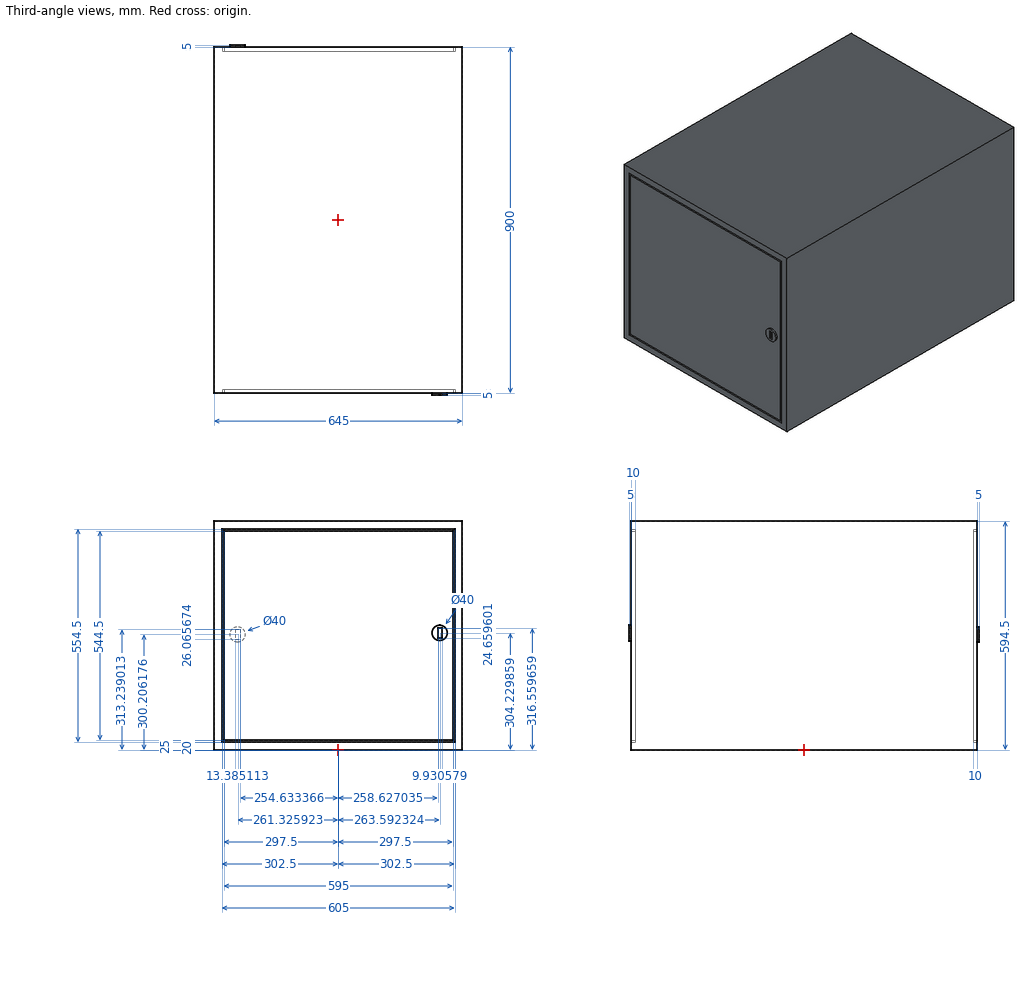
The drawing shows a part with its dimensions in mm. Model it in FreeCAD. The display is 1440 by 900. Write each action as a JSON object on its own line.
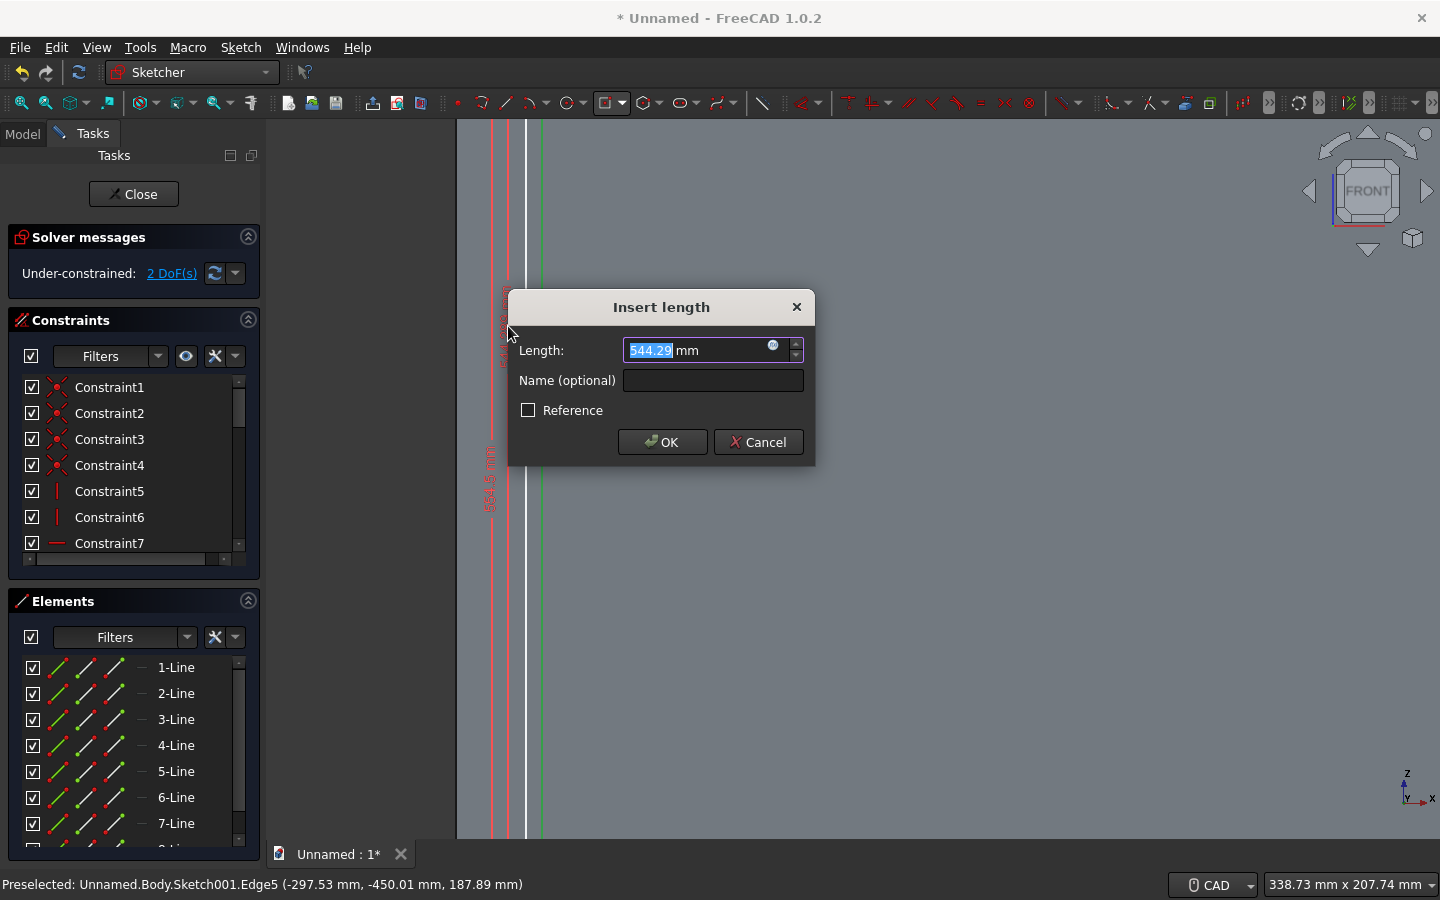
{"action": "type", "text": "544.5"}
{"action": "key", "text": "Return"}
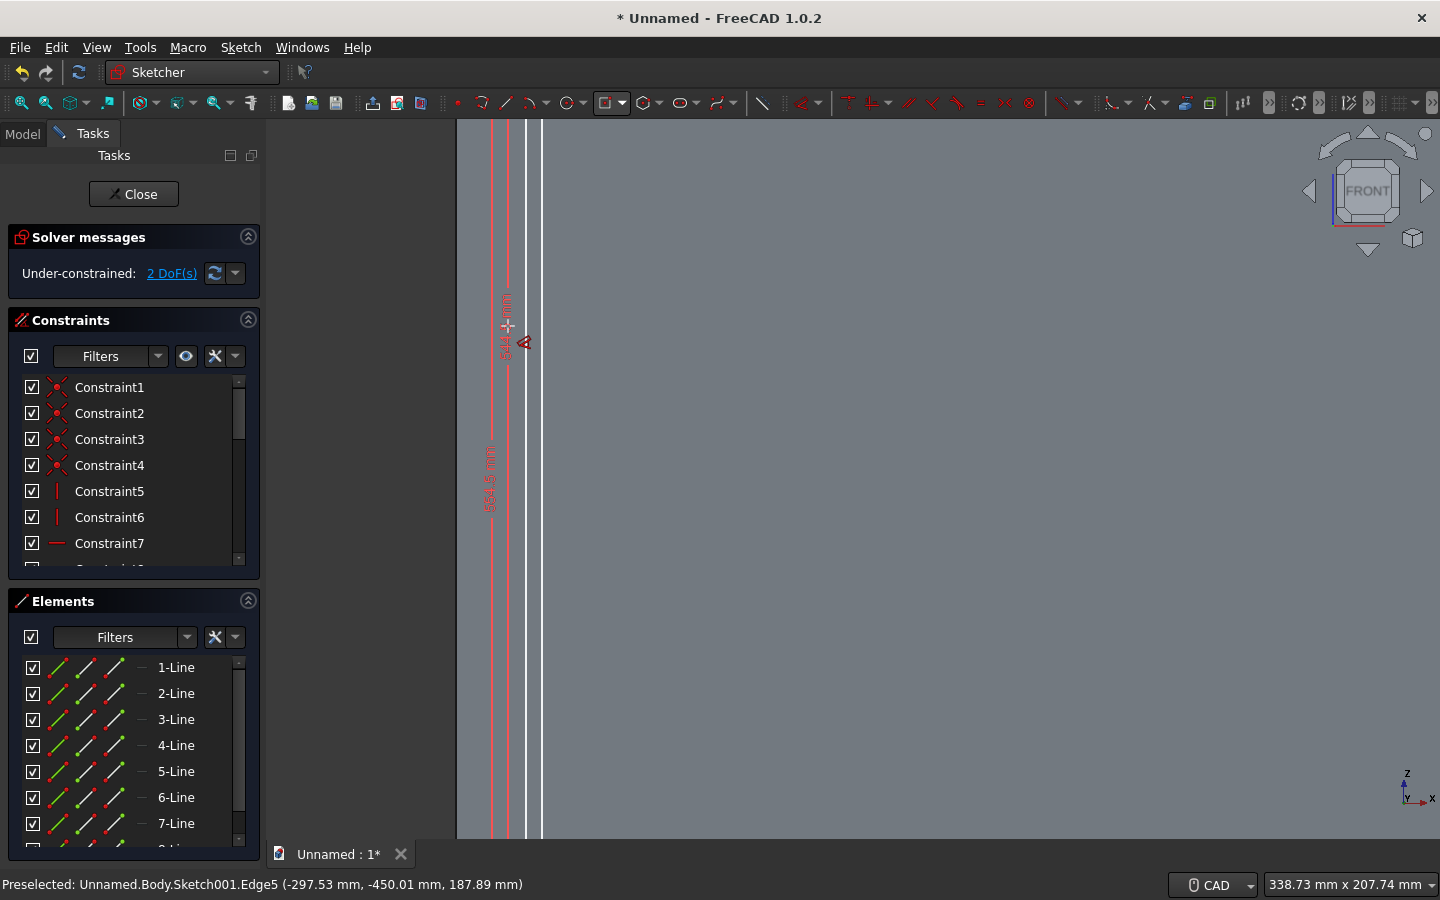
{"action": "scroll", "coordinate": [526, 646], "scroll_direction": "down", "scroll_amount": 7}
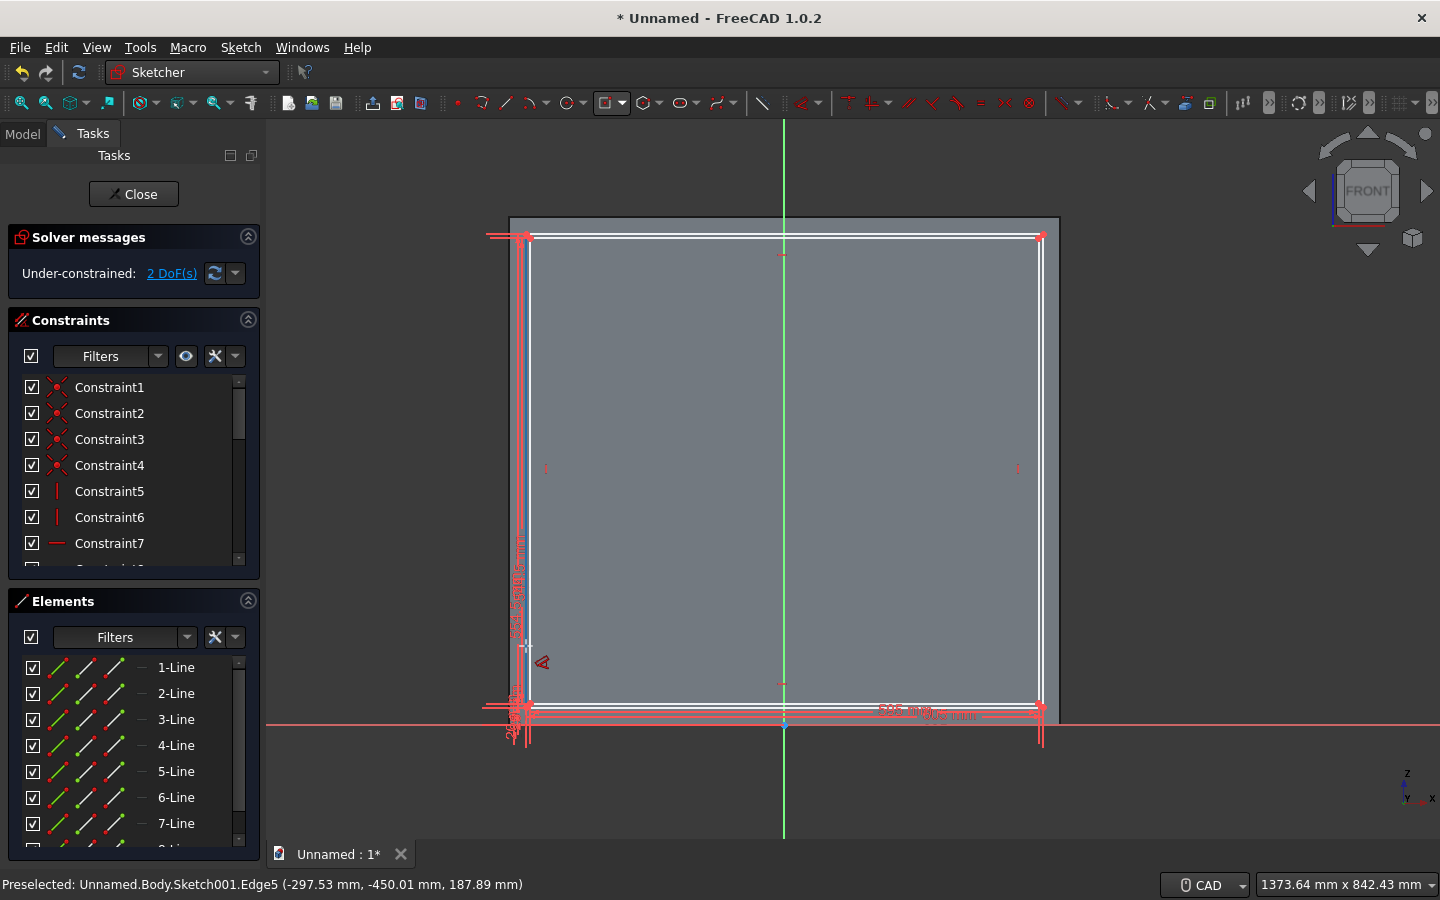
{"action": "scroll", "coordinate": [526, 234], "scroll_direction": "up", "scroll_amount": 4}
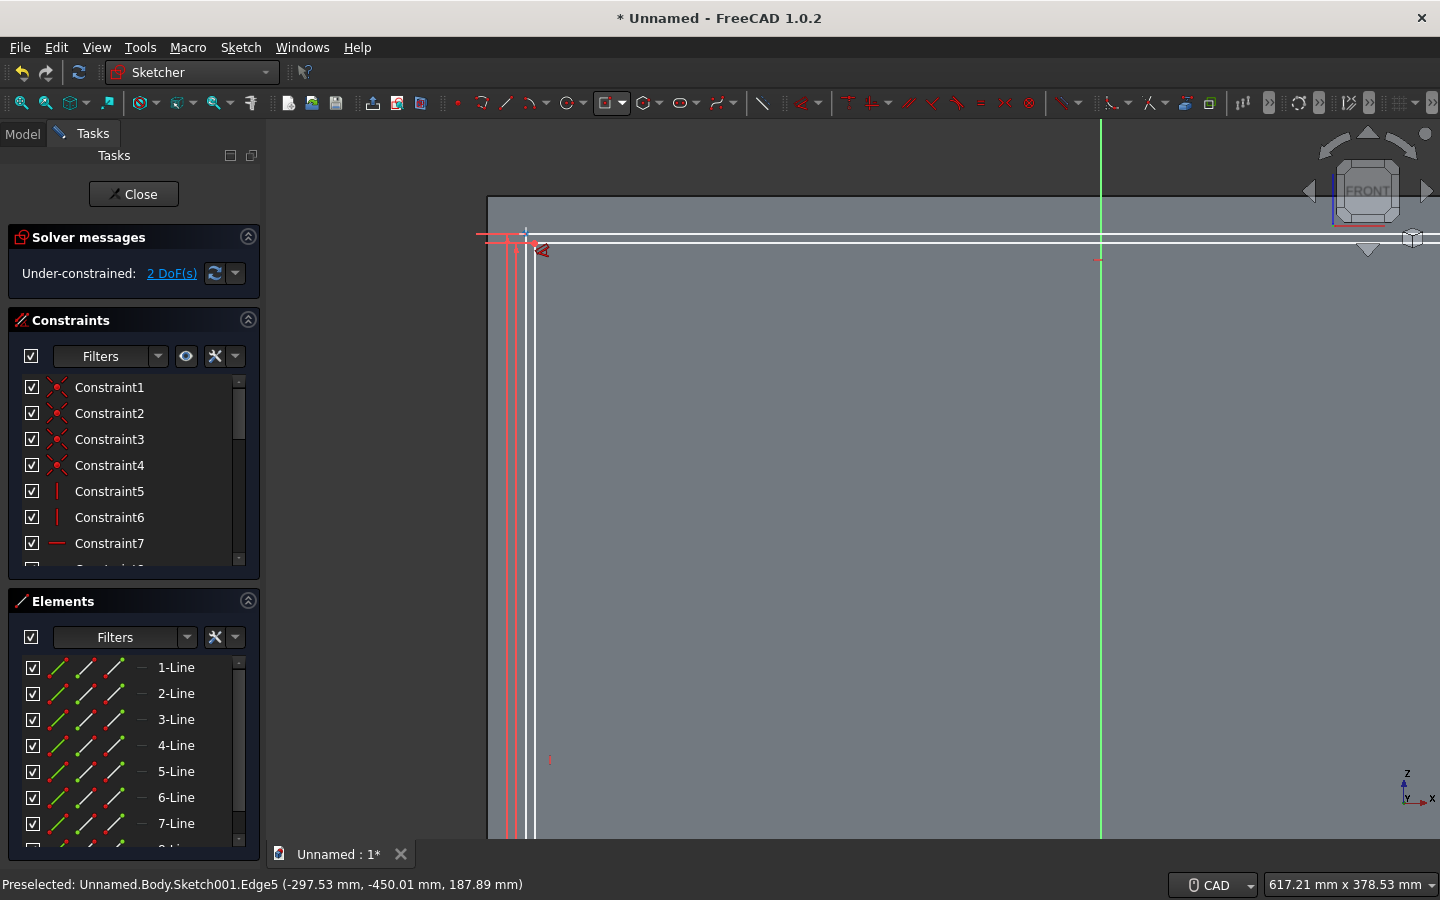
{"action": "left_click", "coordinate": [526, 234]}
{"action": "left_click", "coordinate": [813, 200]}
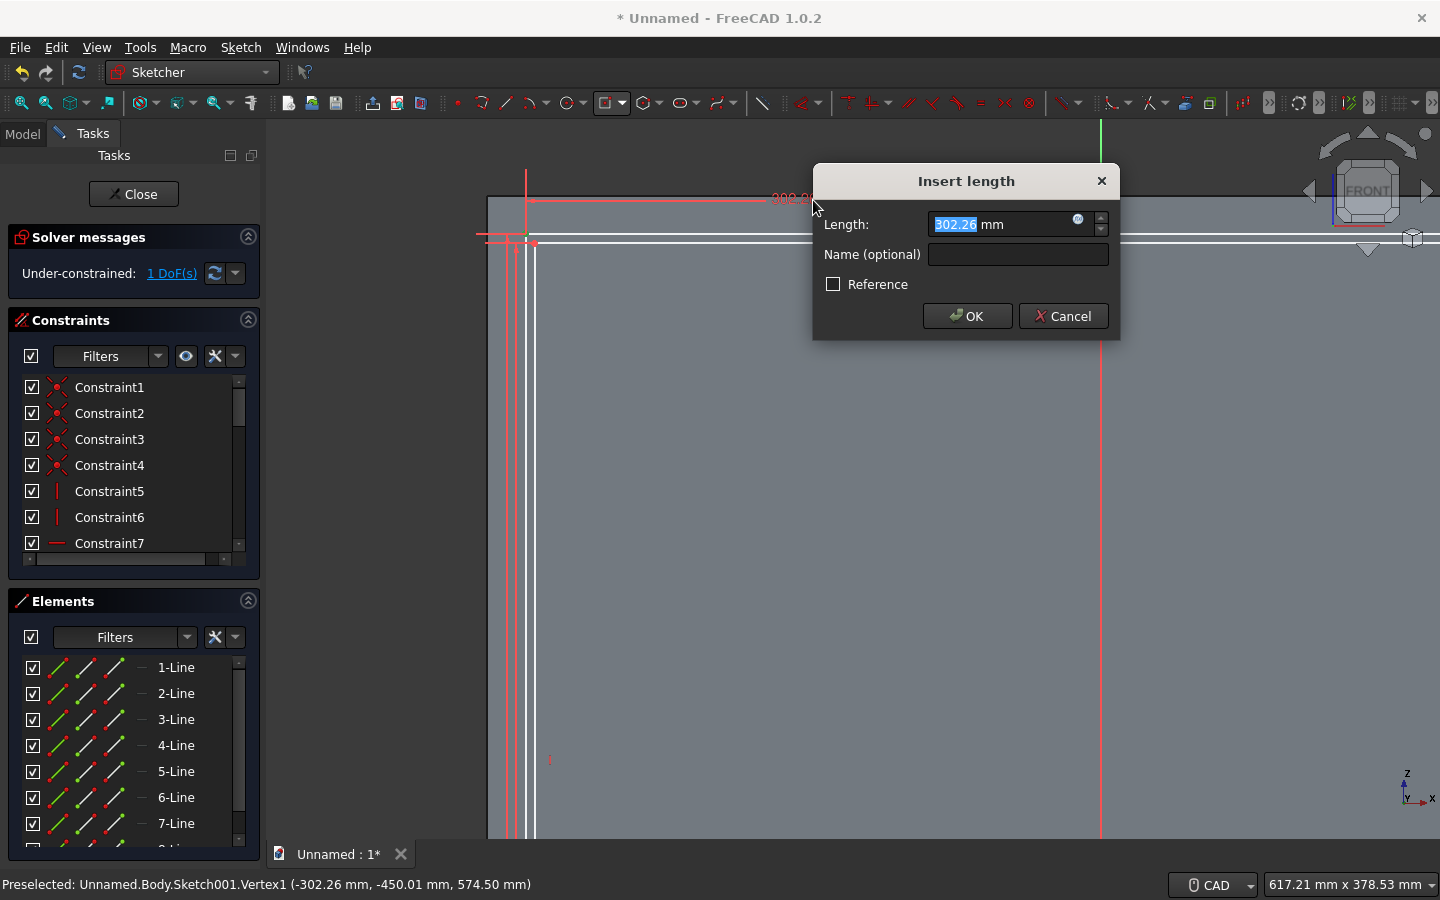
{"action": "type", "text": "302.5"}
{"action": "key", "text": "Return"}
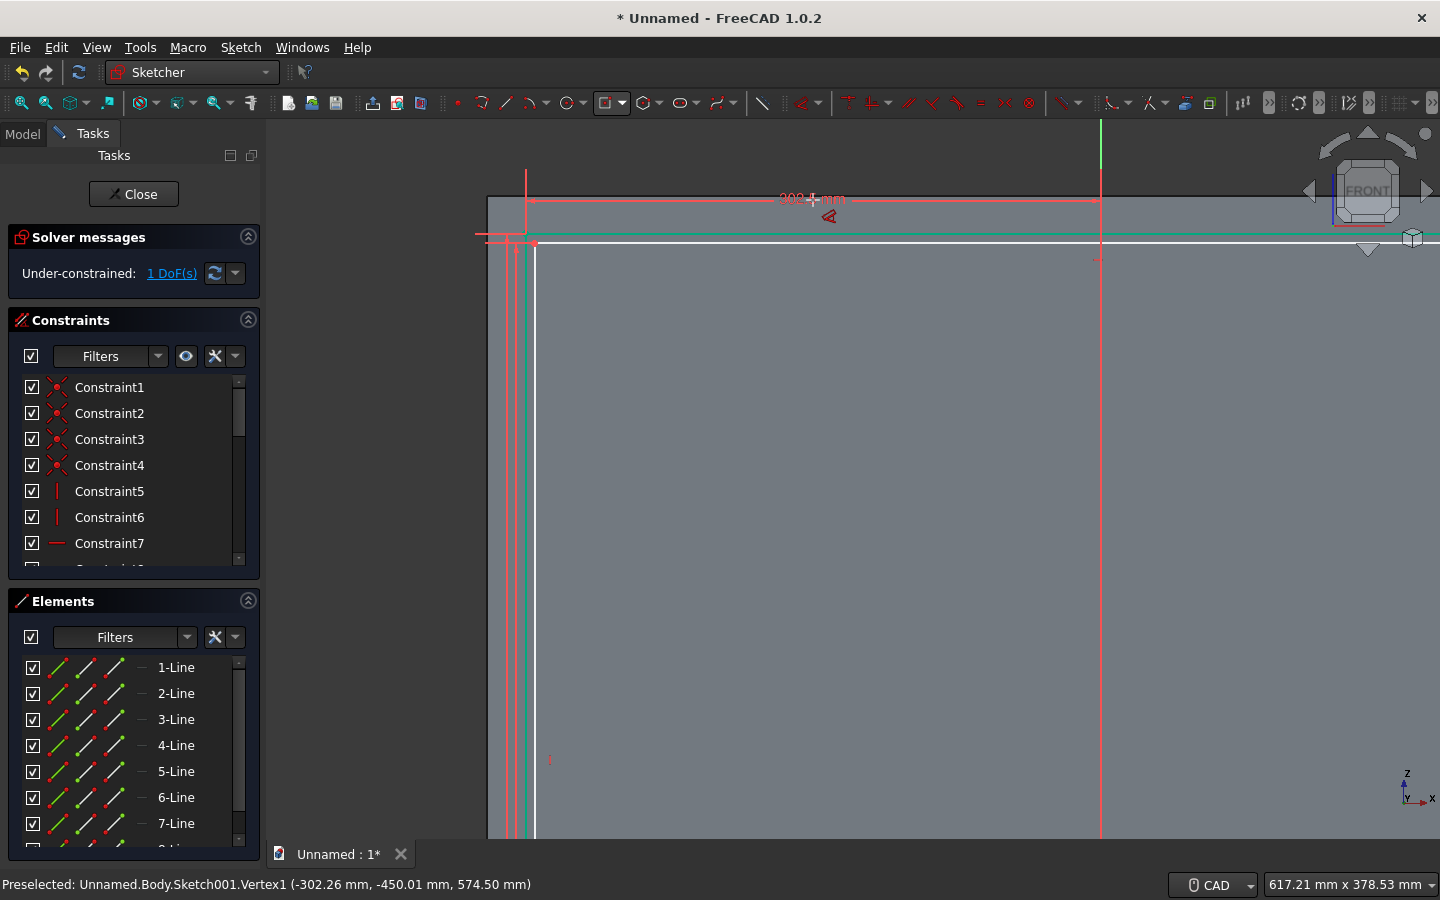
{"action": "left_click", "coordinate": [535, 243]}
{"action": "left_click", "coordinate": [688, 209]}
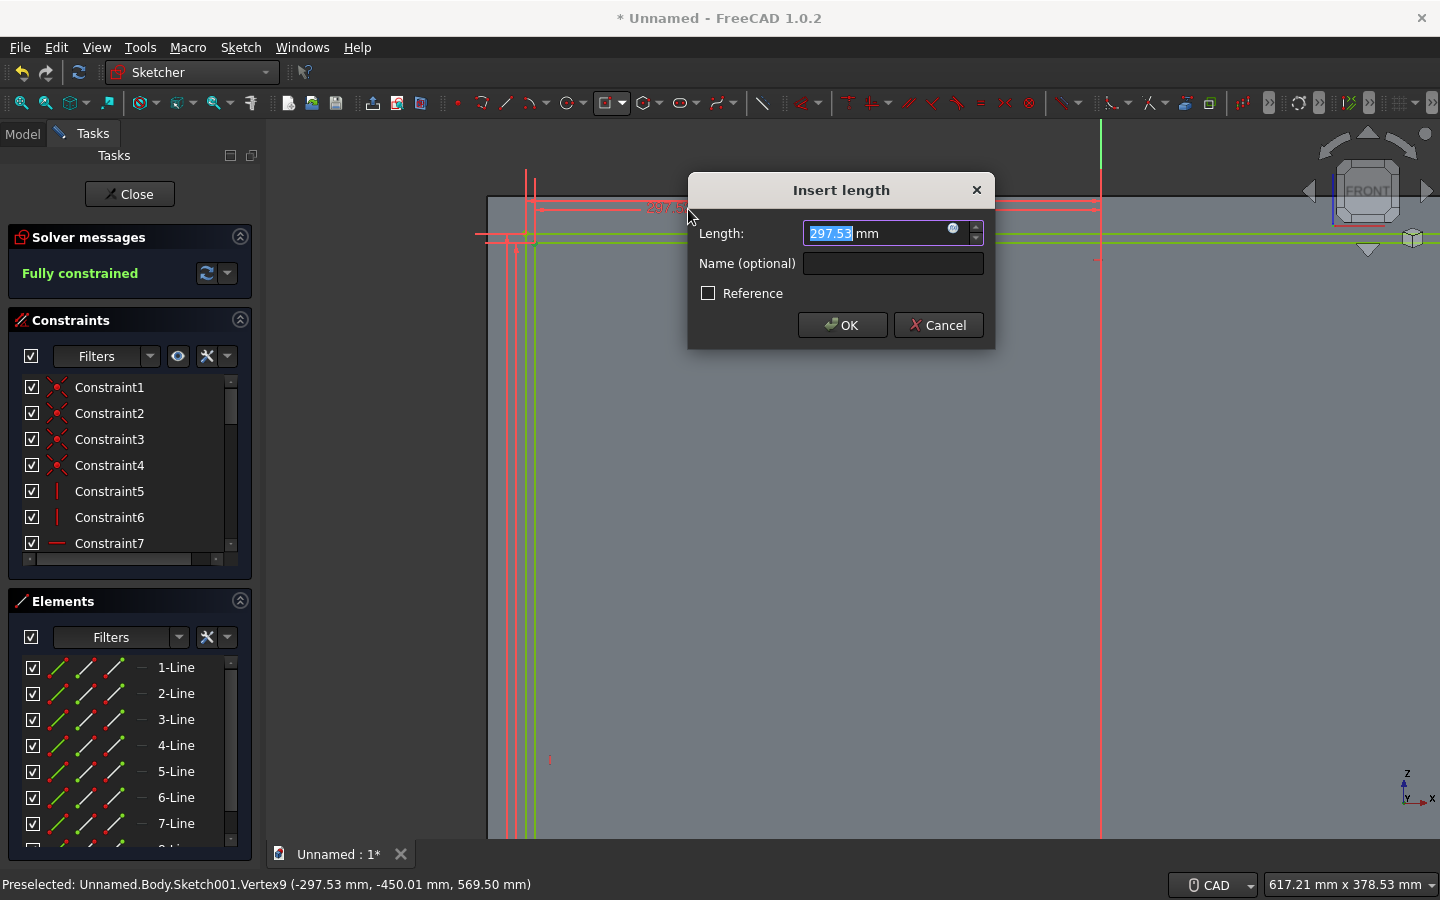
{"action": "type", "text": "297.5"}
{"action": "key", "text": "Return"}
{"action": "key", "text": "Escape"}